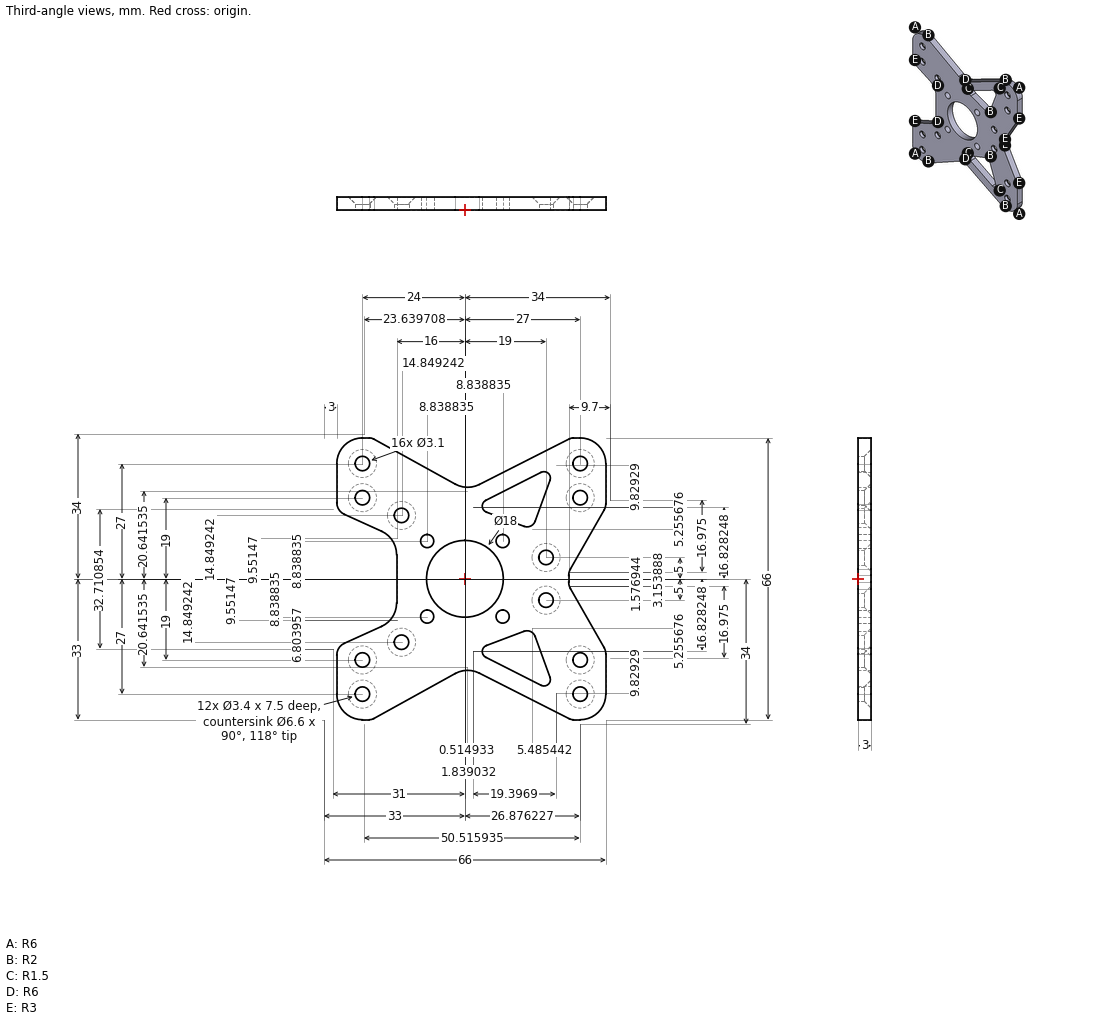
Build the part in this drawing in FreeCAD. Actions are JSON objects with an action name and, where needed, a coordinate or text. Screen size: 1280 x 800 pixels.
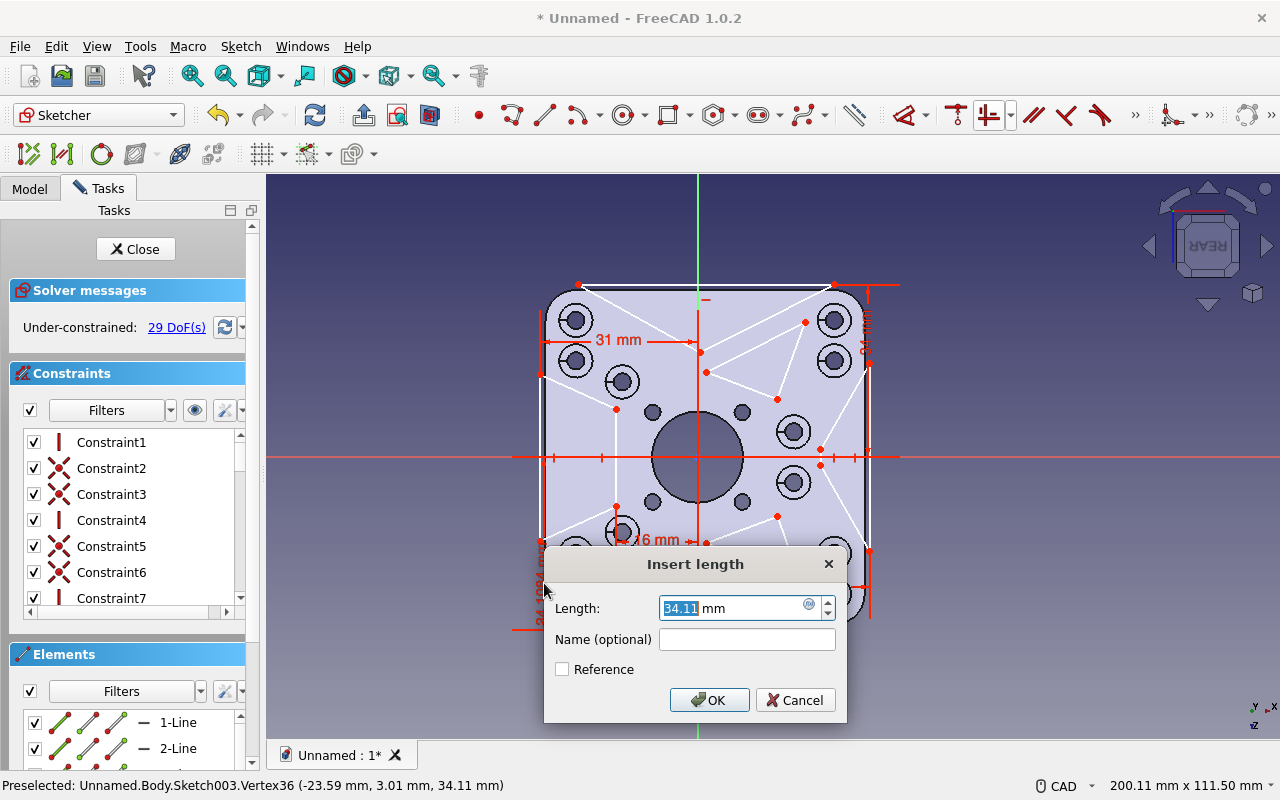
{"action": "type", "text": "34"}
{"action": "key", "text": "Return"}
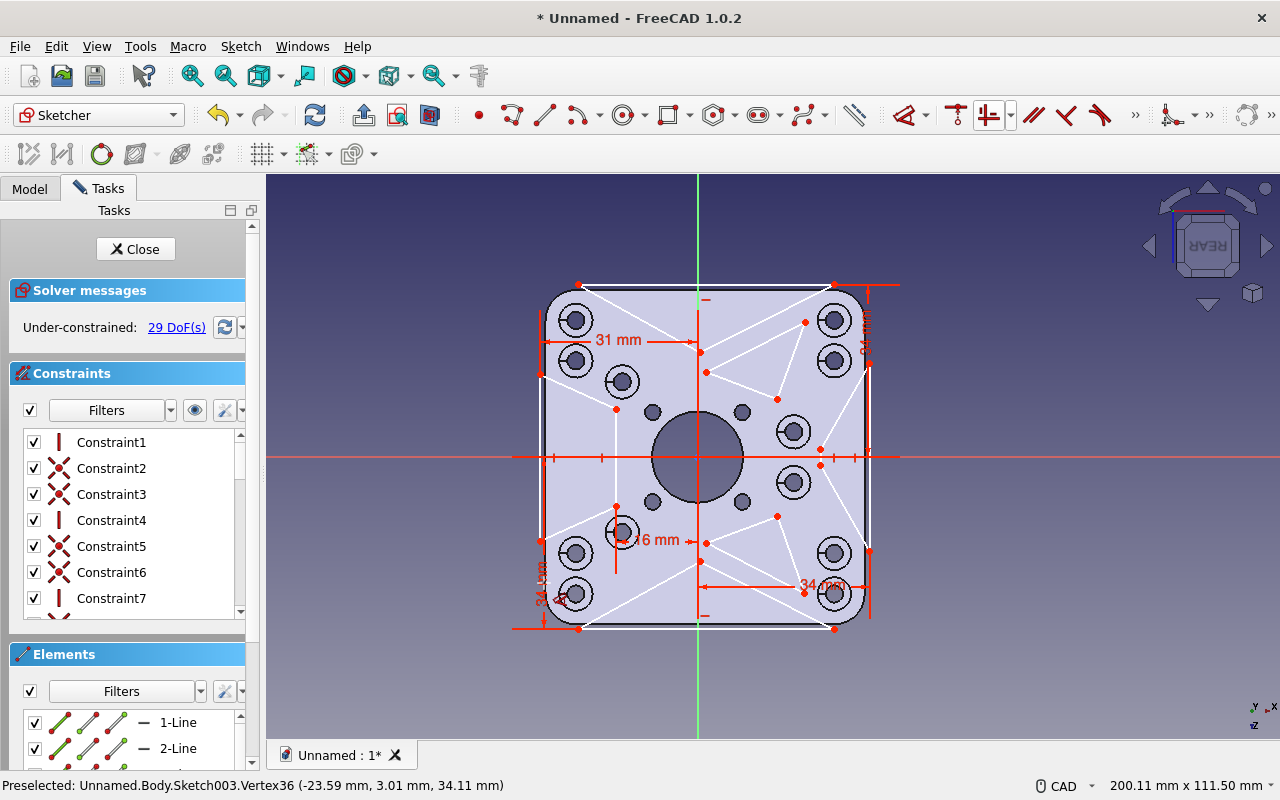
{"action": "left_click", "coordinate": [835, 491]}
{"action": "left_click", "coordinate": [857, 432]}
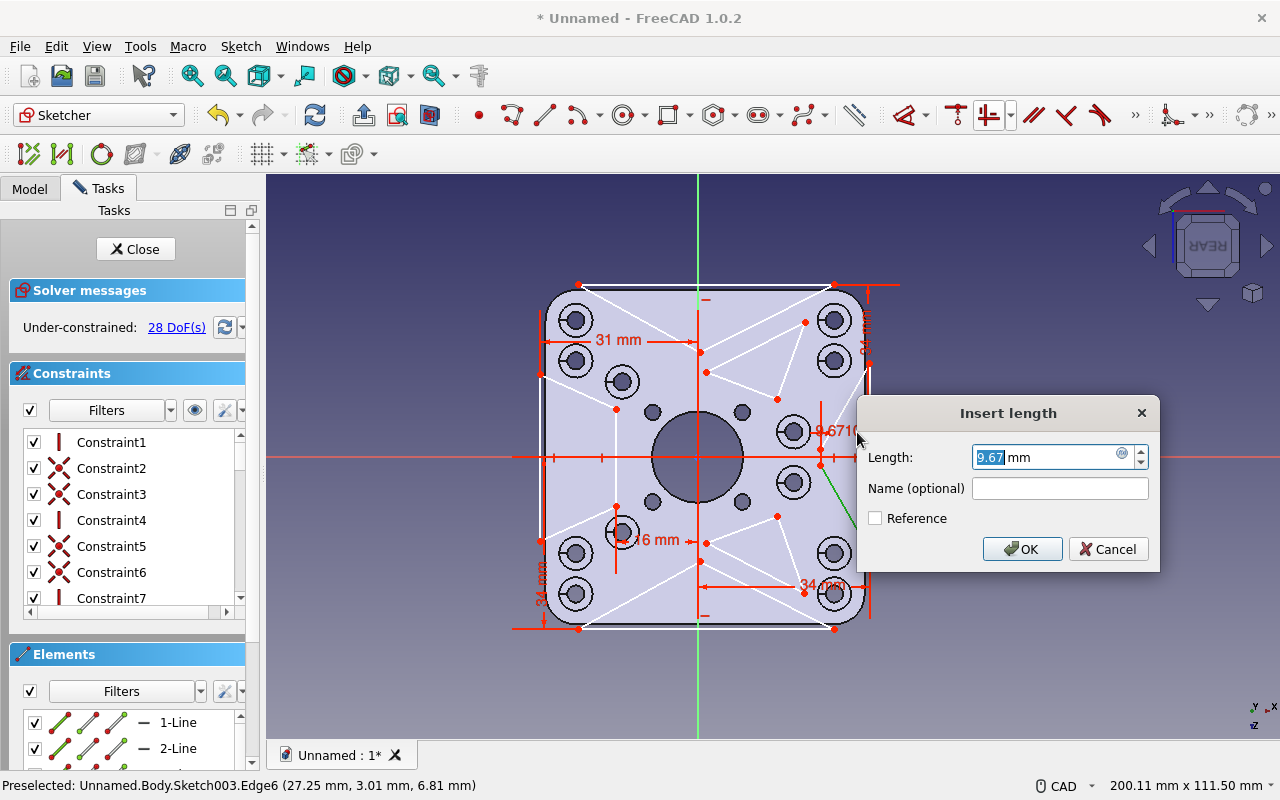
{"action": "type", "text": "9.7"}
{"action": "key", "text": "Return"}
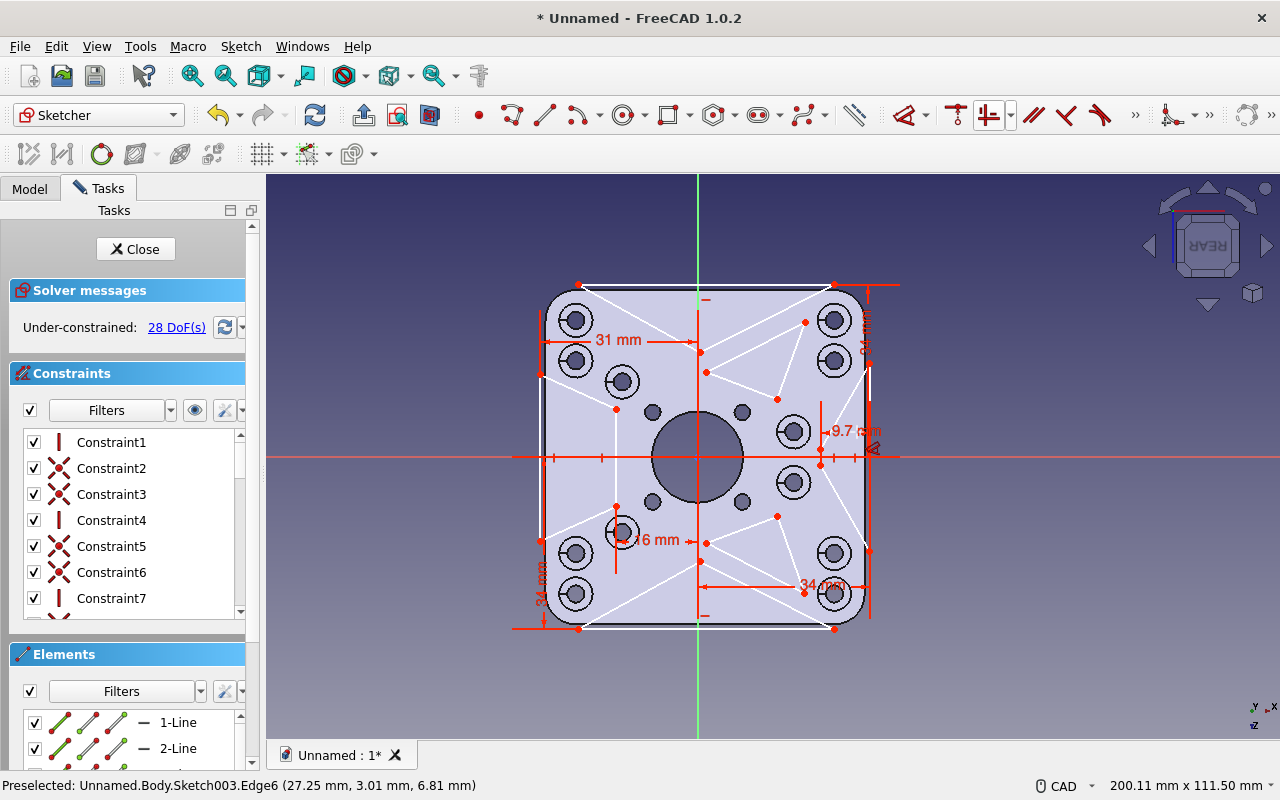
{"action": "left_click", "coordinate": [835, 491]}
{"action": "left_click", "coordinate": [904, 509]}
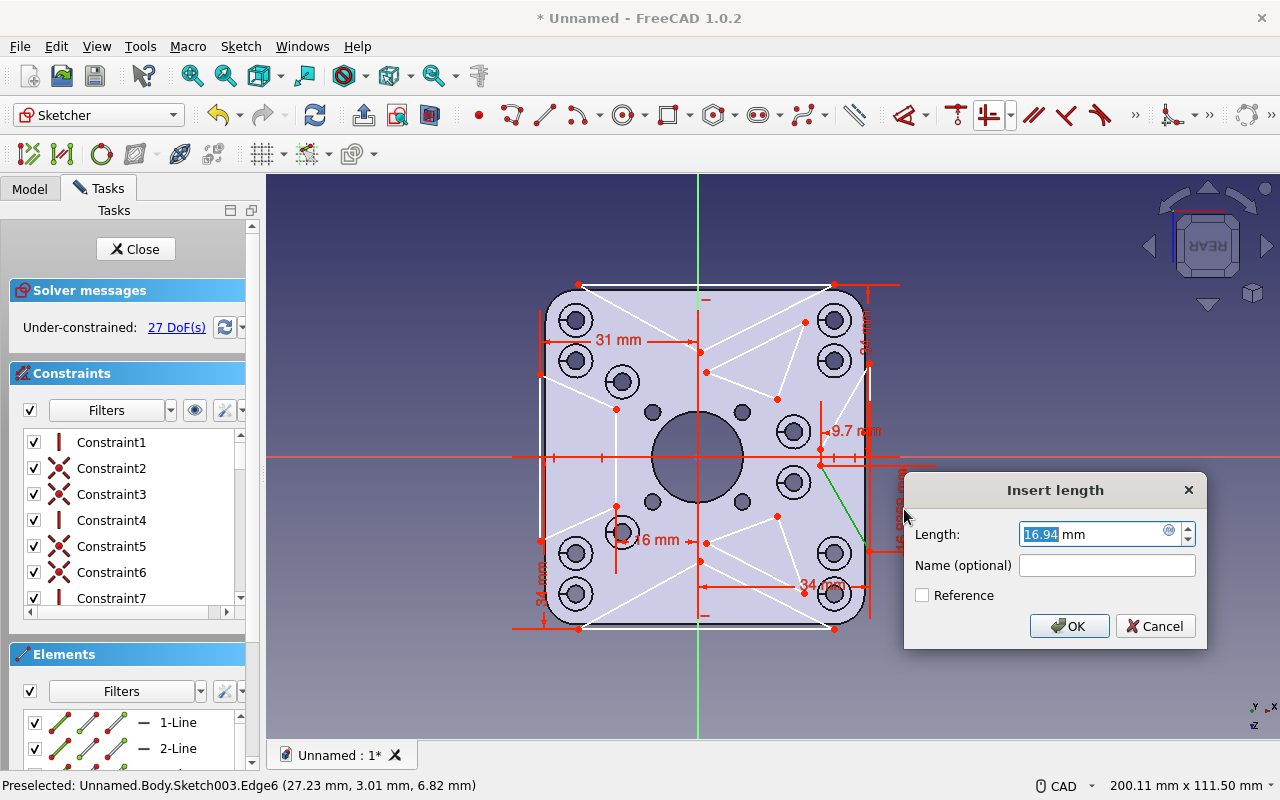
{"action": "type", "text": "16.975"}
{"action": "key", "text": "Return"}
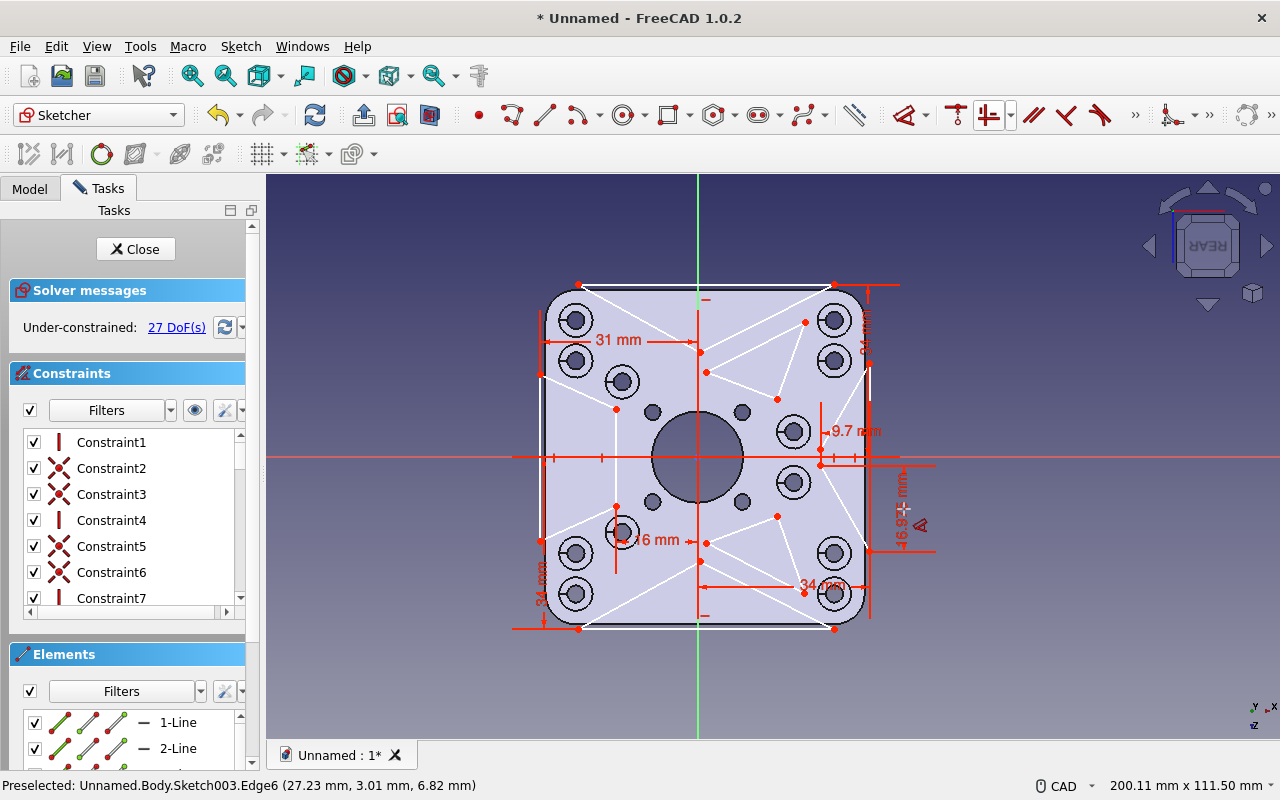
{"action": "left_click", "coordinate": [855, 389]}
{"action": "left_click", "coordinate": [904, 407]}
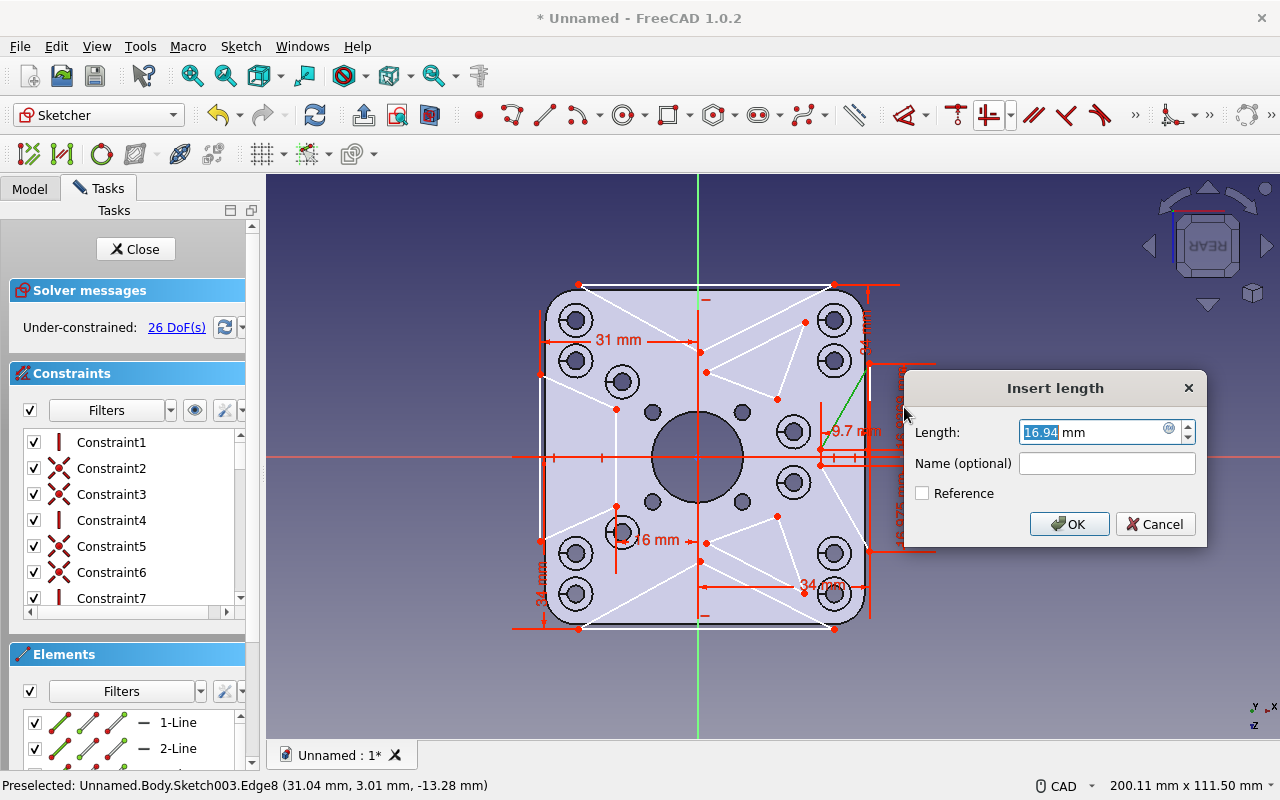
{"action": "type", "text": "16.975"}
{"action": "key", "text": "Return"}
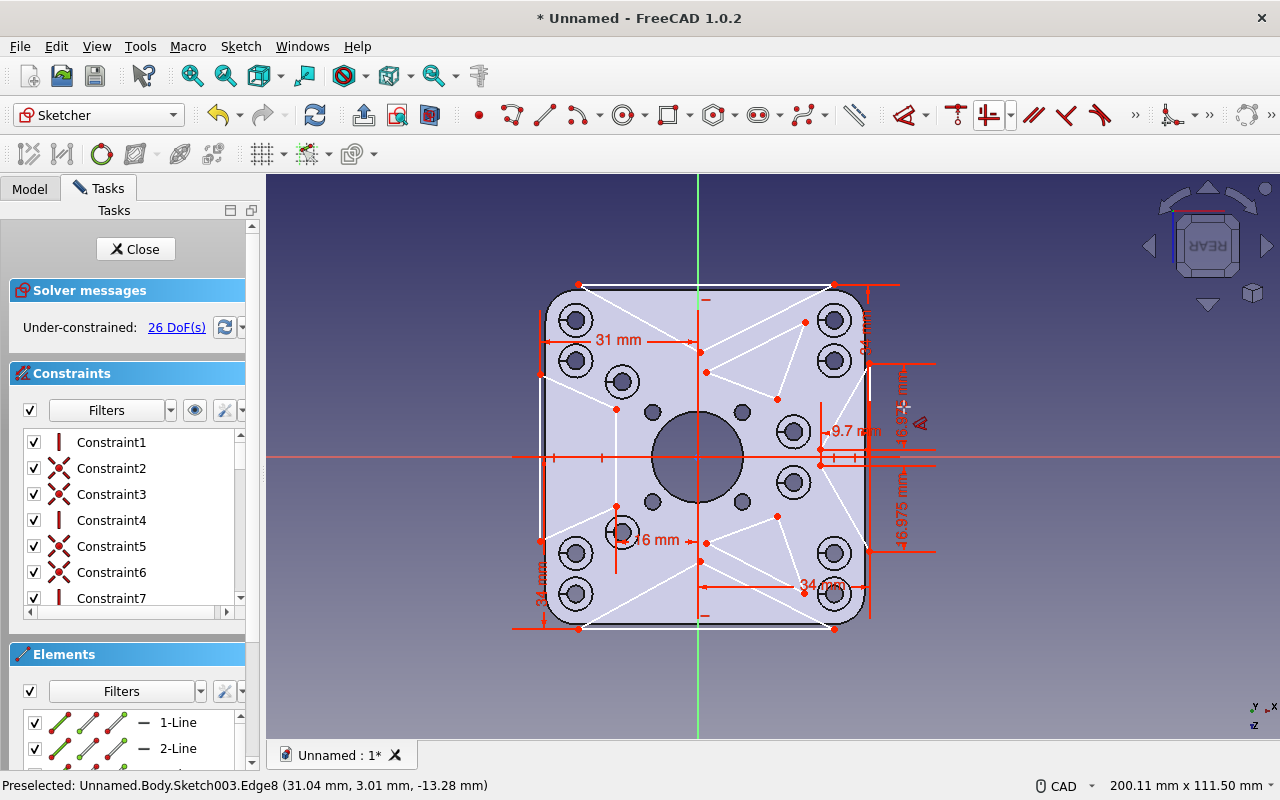
{"action": "scroll", "coordinate": [821, 458], "scroll_direction": "up", "scroll_amount": 5}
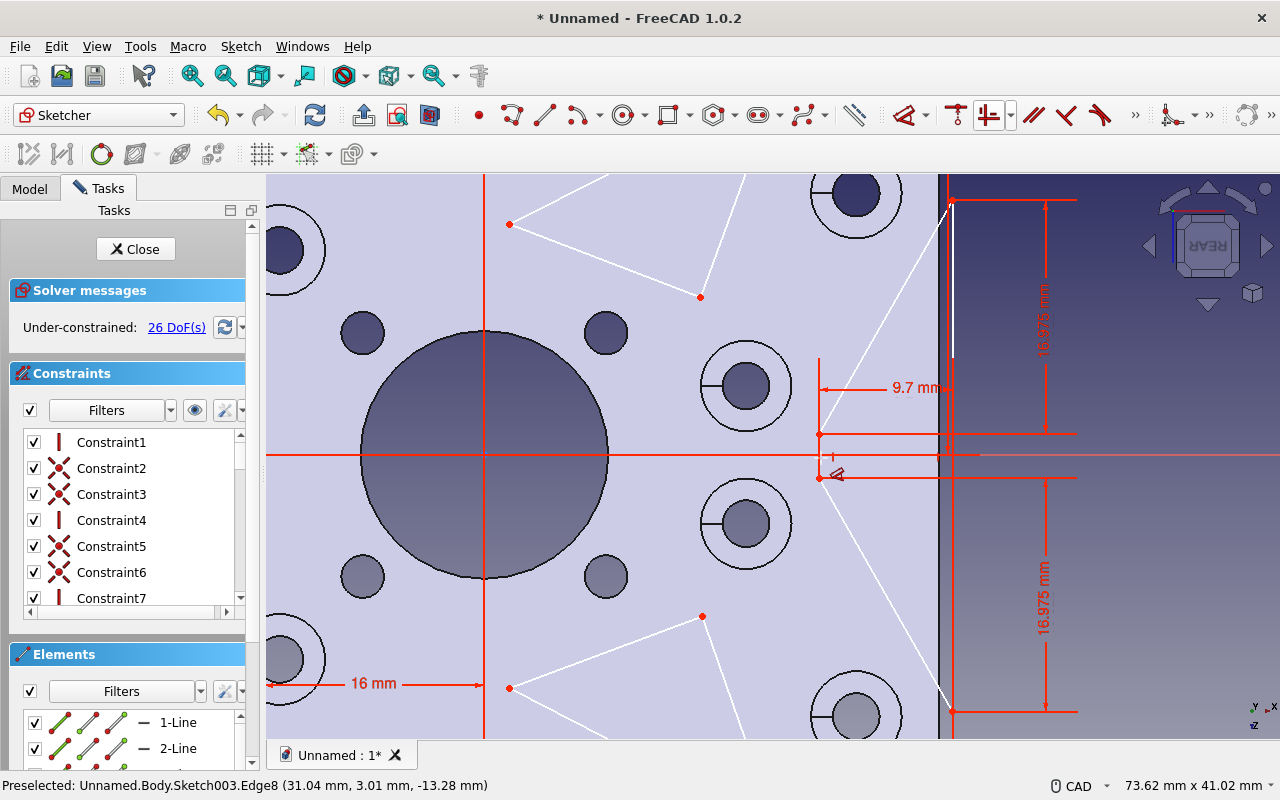
{"action": "left_click", "coordinate": [819, 456]}
{"action": "left_click", "coordinate": [853, 441]}